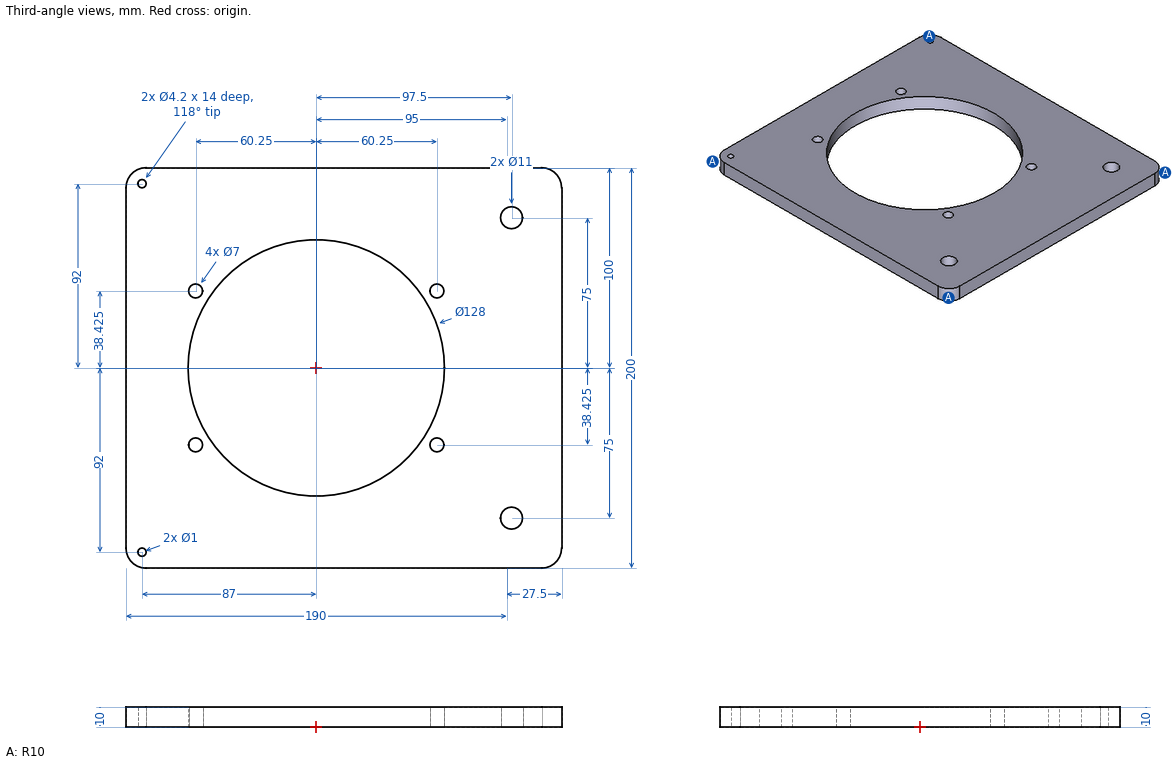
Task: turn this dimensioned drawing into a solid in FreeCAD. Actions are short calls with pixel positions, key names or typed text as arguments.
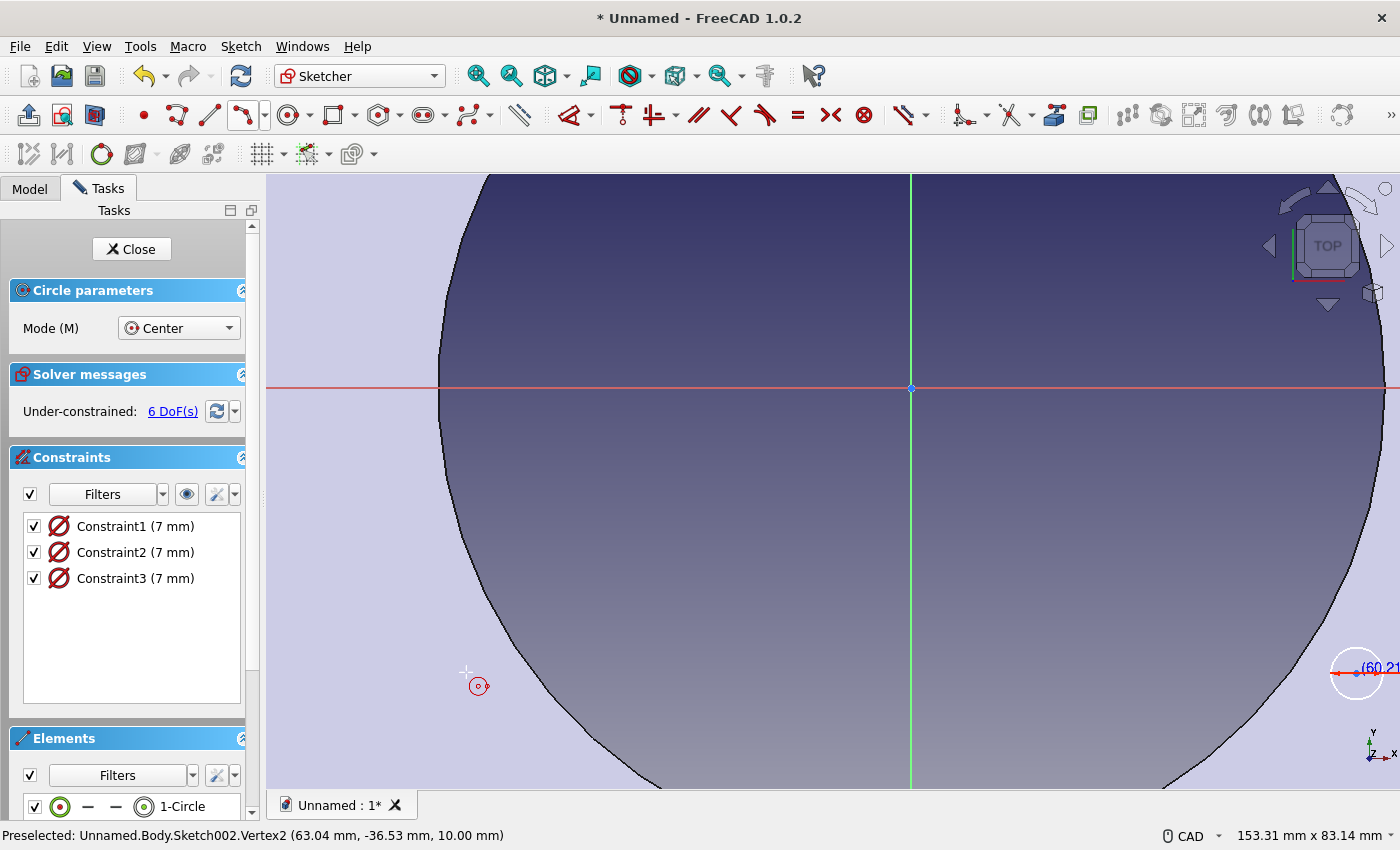
click(466, 672)
move(484, 654)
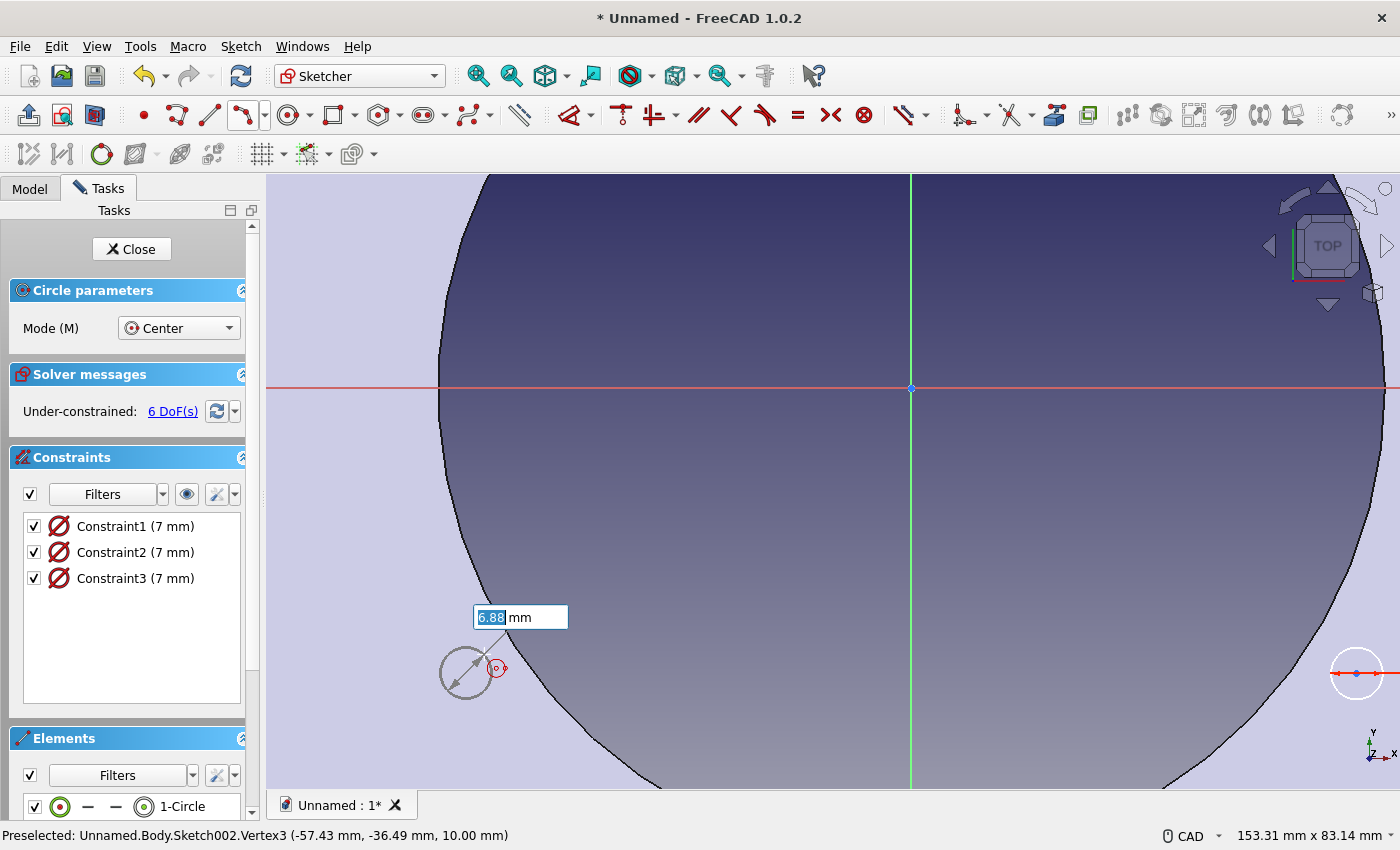
text(7)
key(Return)
key(Escape)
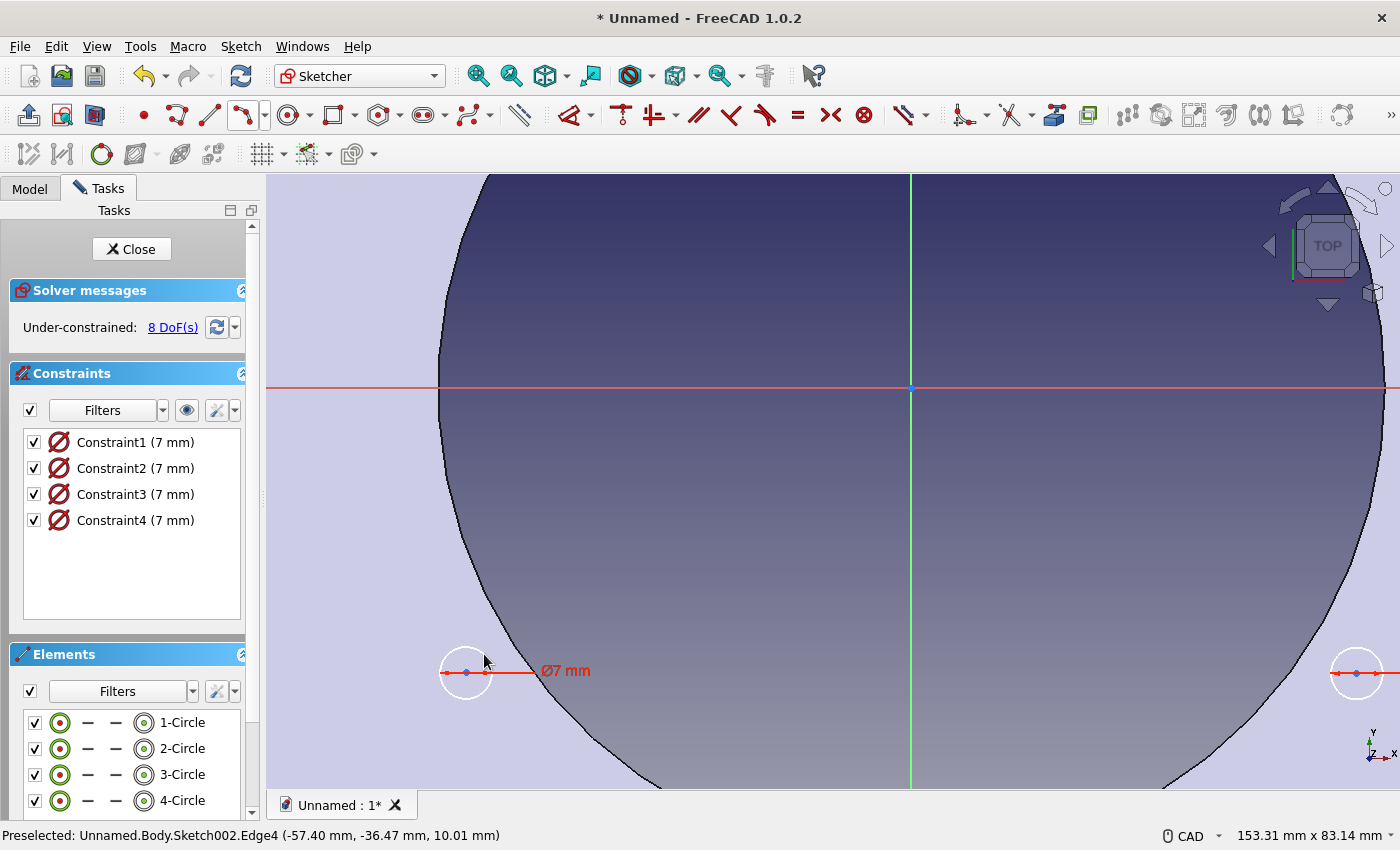
scroll(466, 672, down, 2)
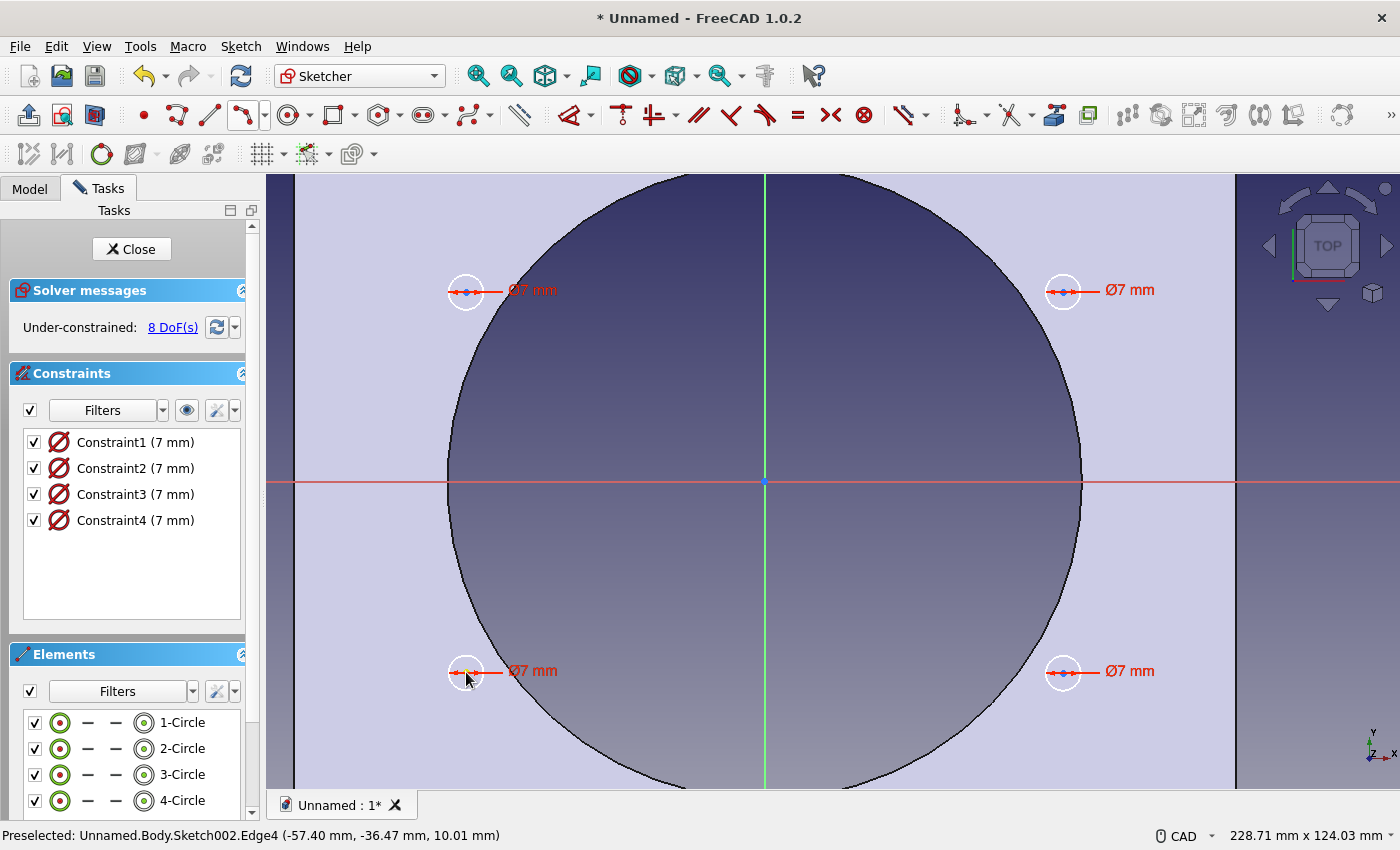
click(466, 292)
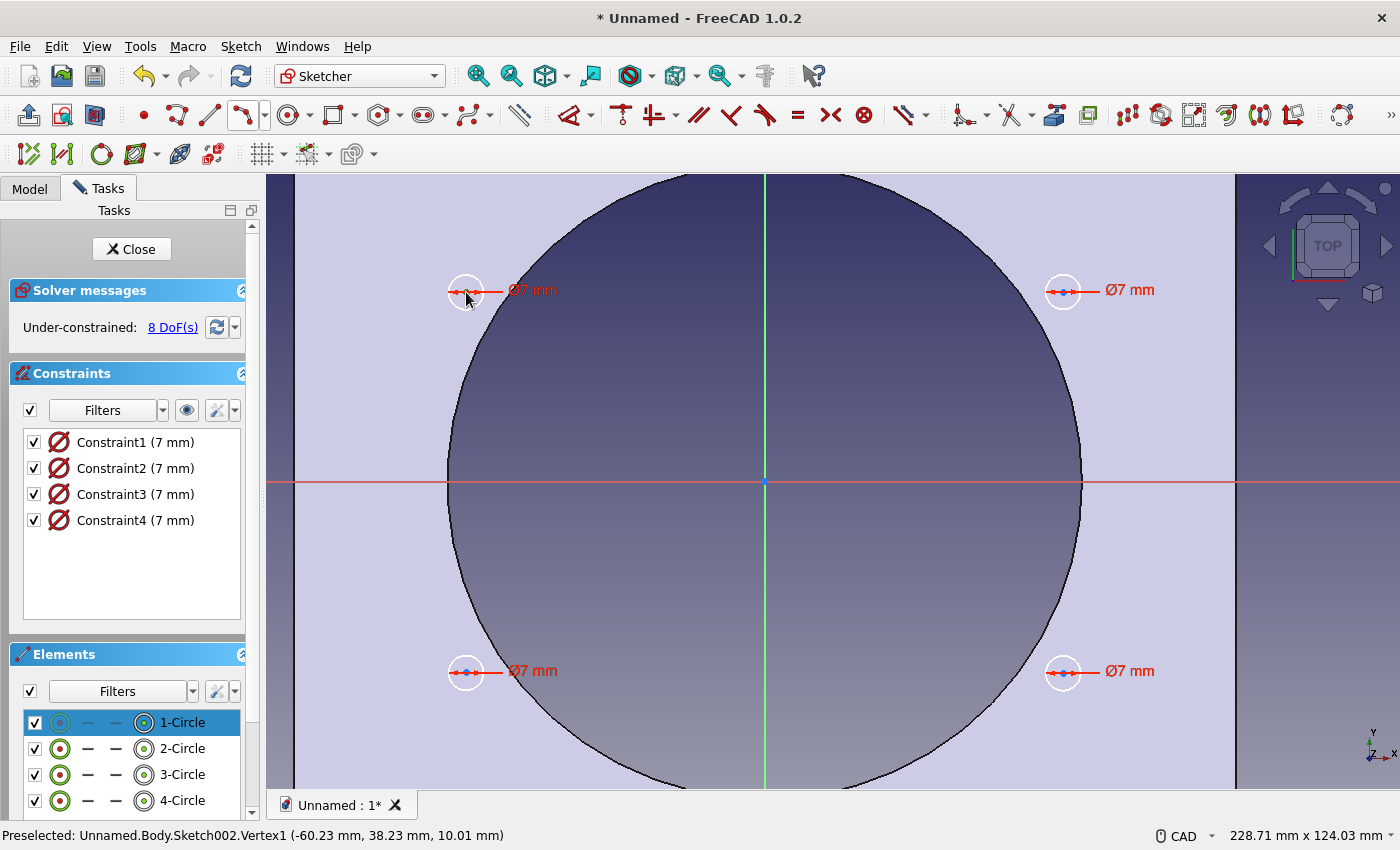
click(1063, 292)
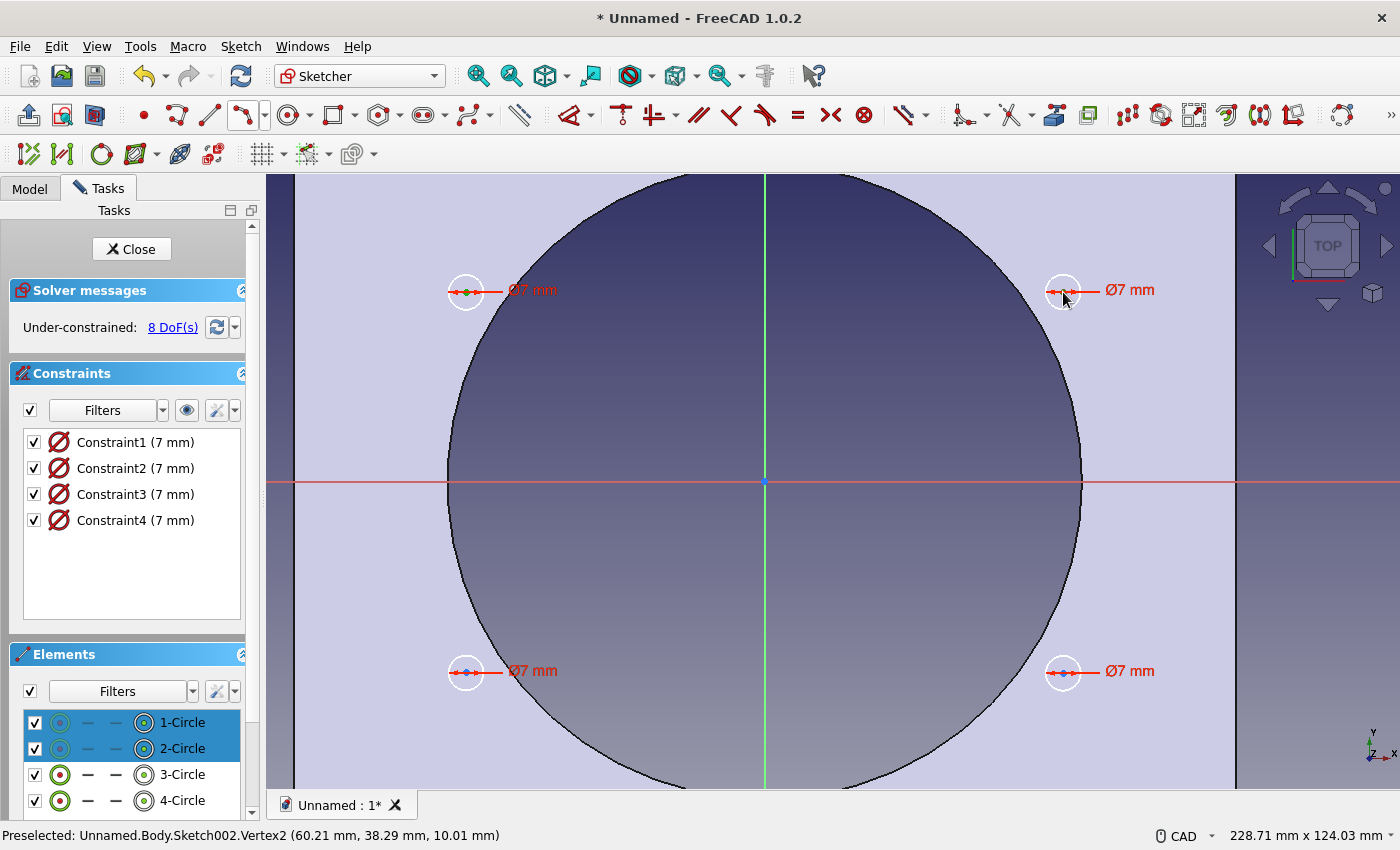
key(h)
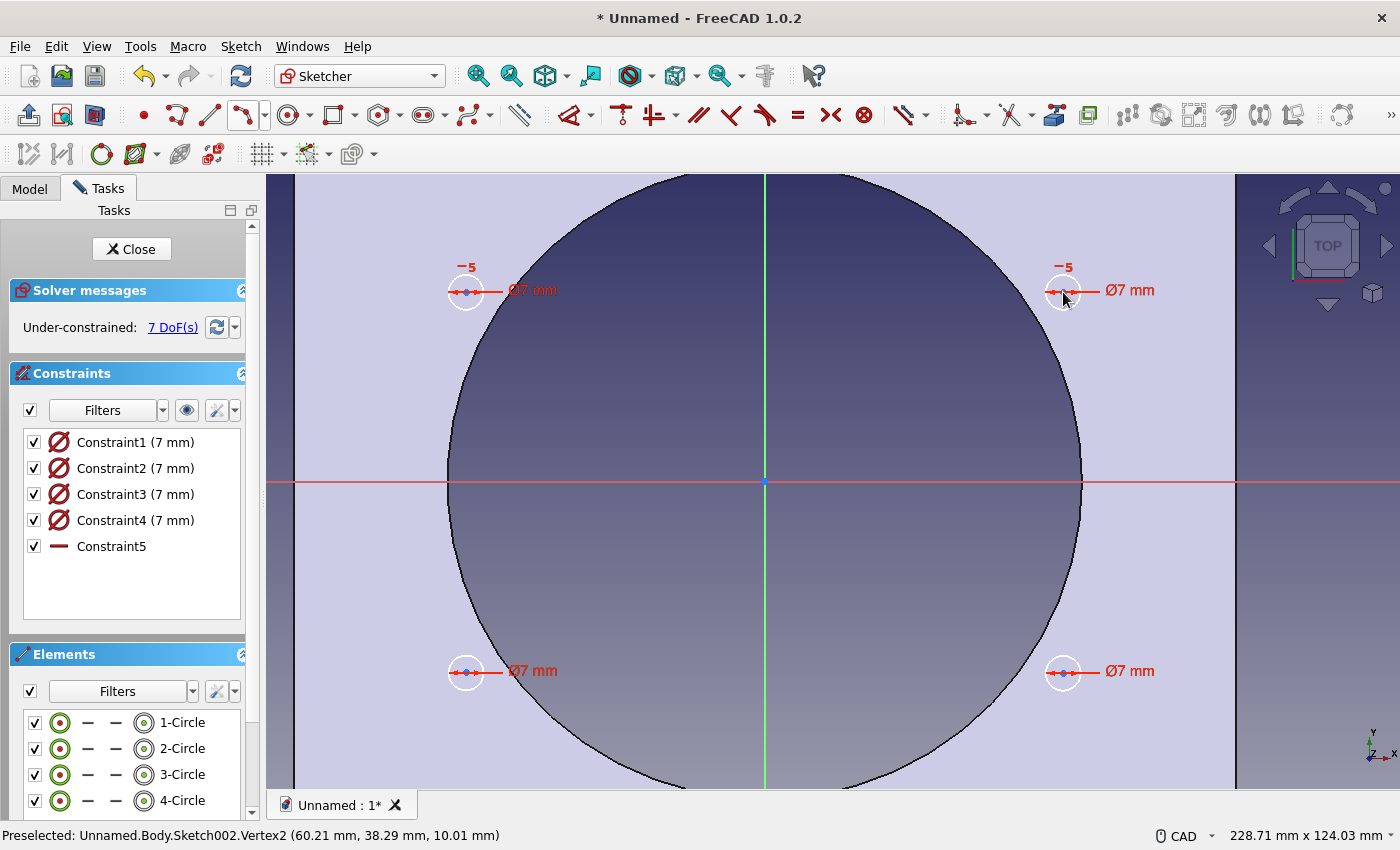
click(1063, 292)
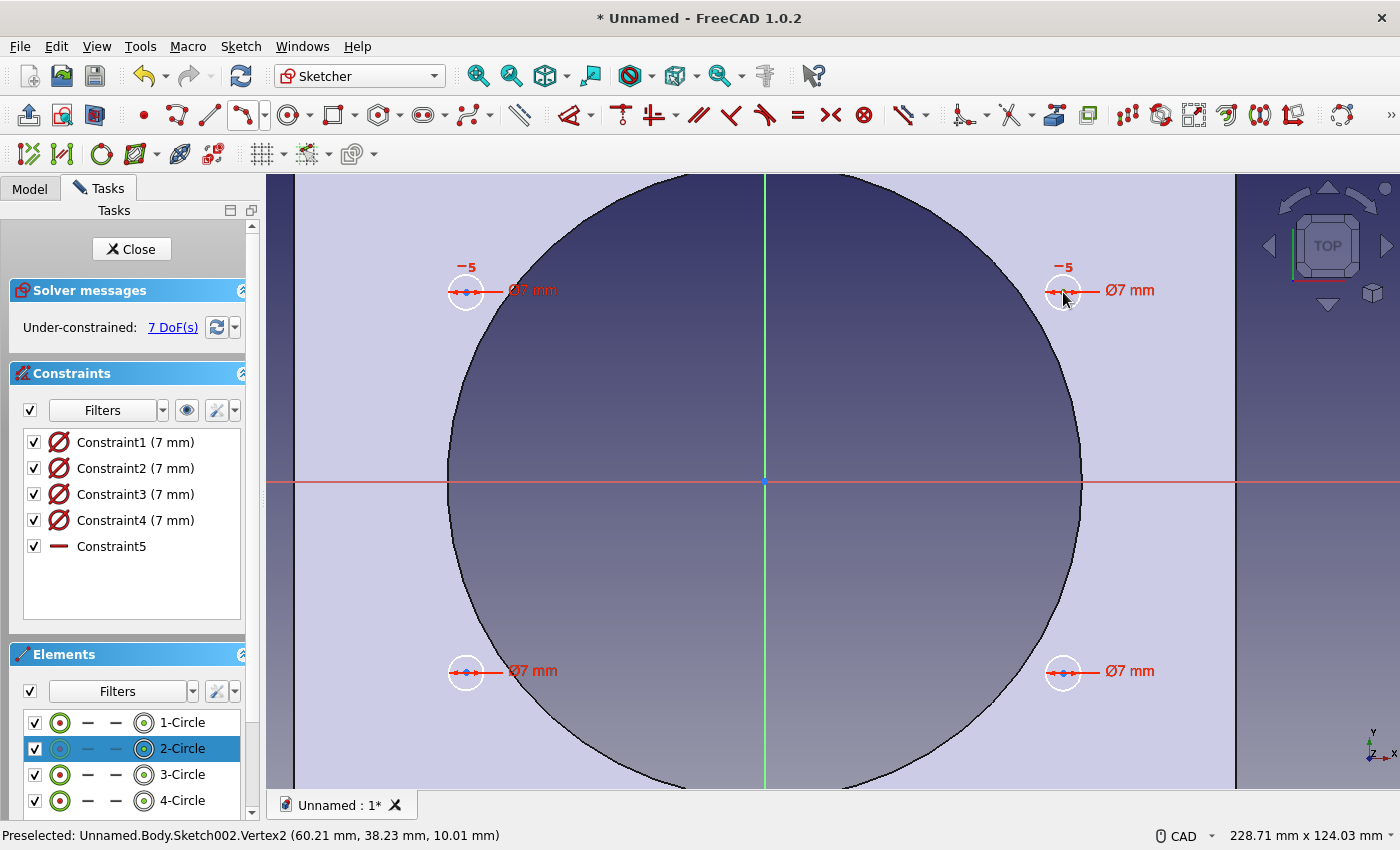
click(1063, 673)